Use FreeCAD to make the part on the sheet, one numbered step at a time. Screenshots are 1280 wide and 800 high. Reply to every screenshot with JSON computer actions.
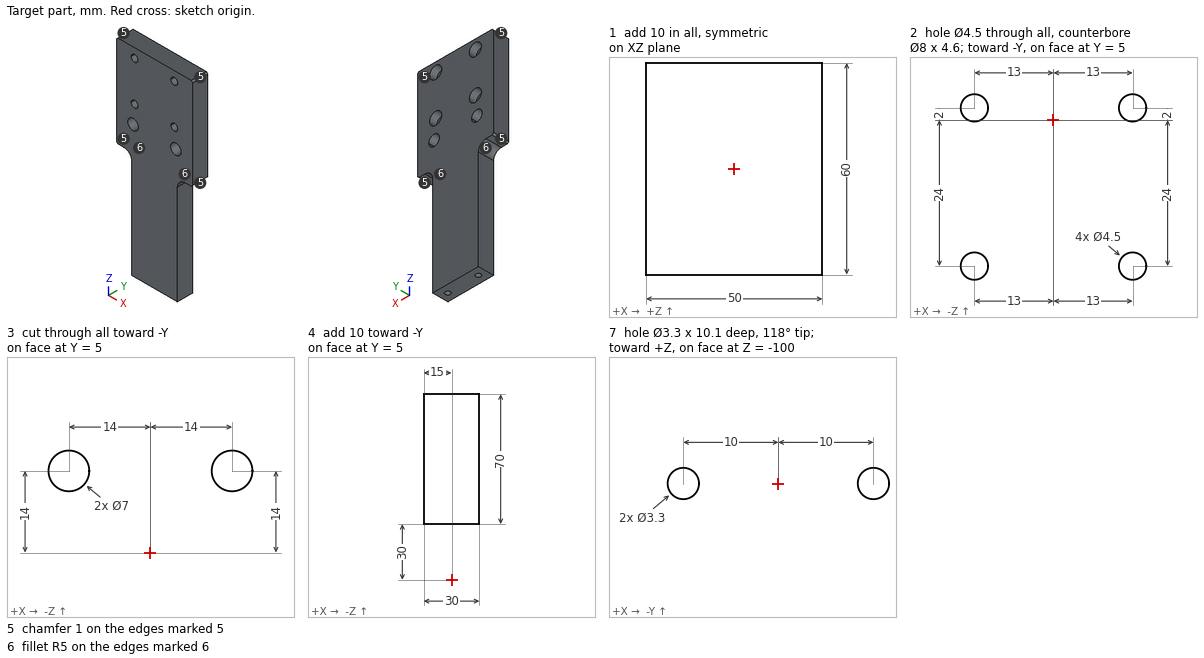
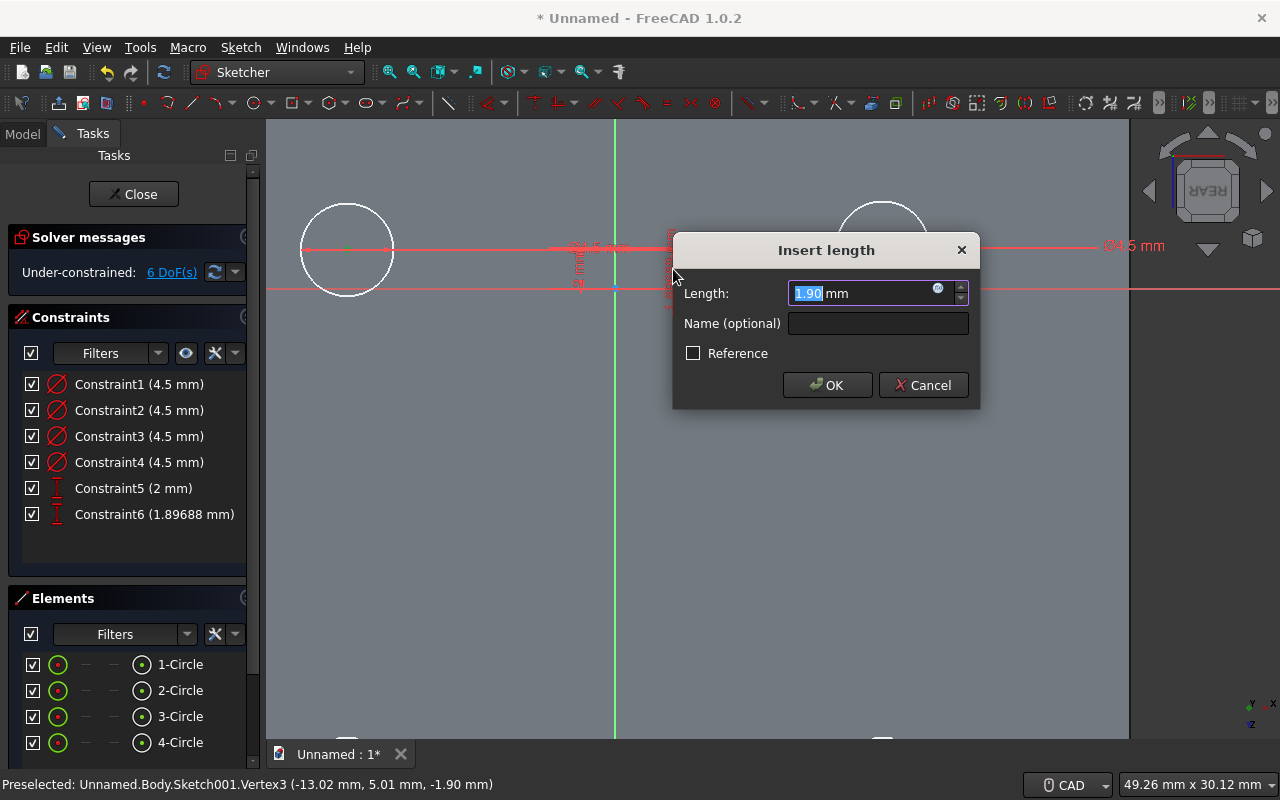
{"action": "type", "text": "2"}
{"action": "key", "text": "Return"}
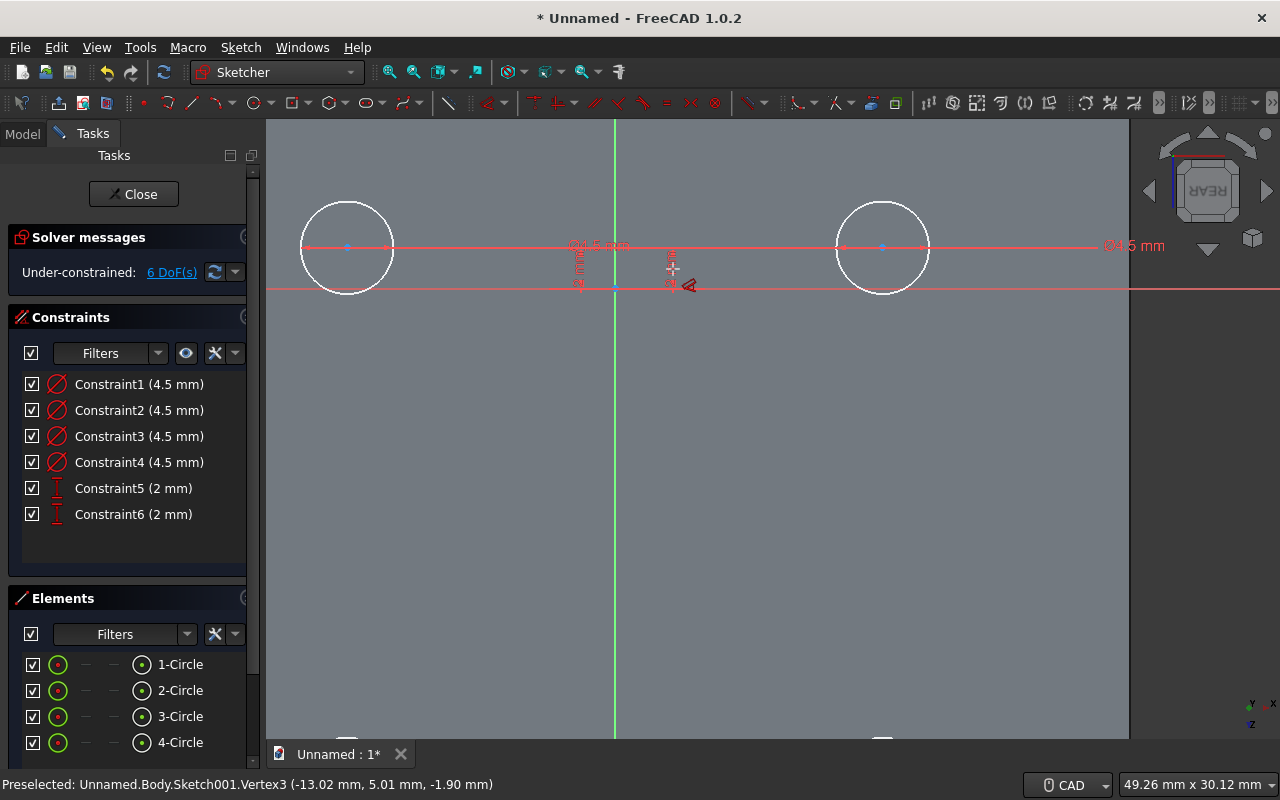
{"action": "scroll", "coordinate": [886, 253], "scroll_direction": "down", "scroll_amount": 2}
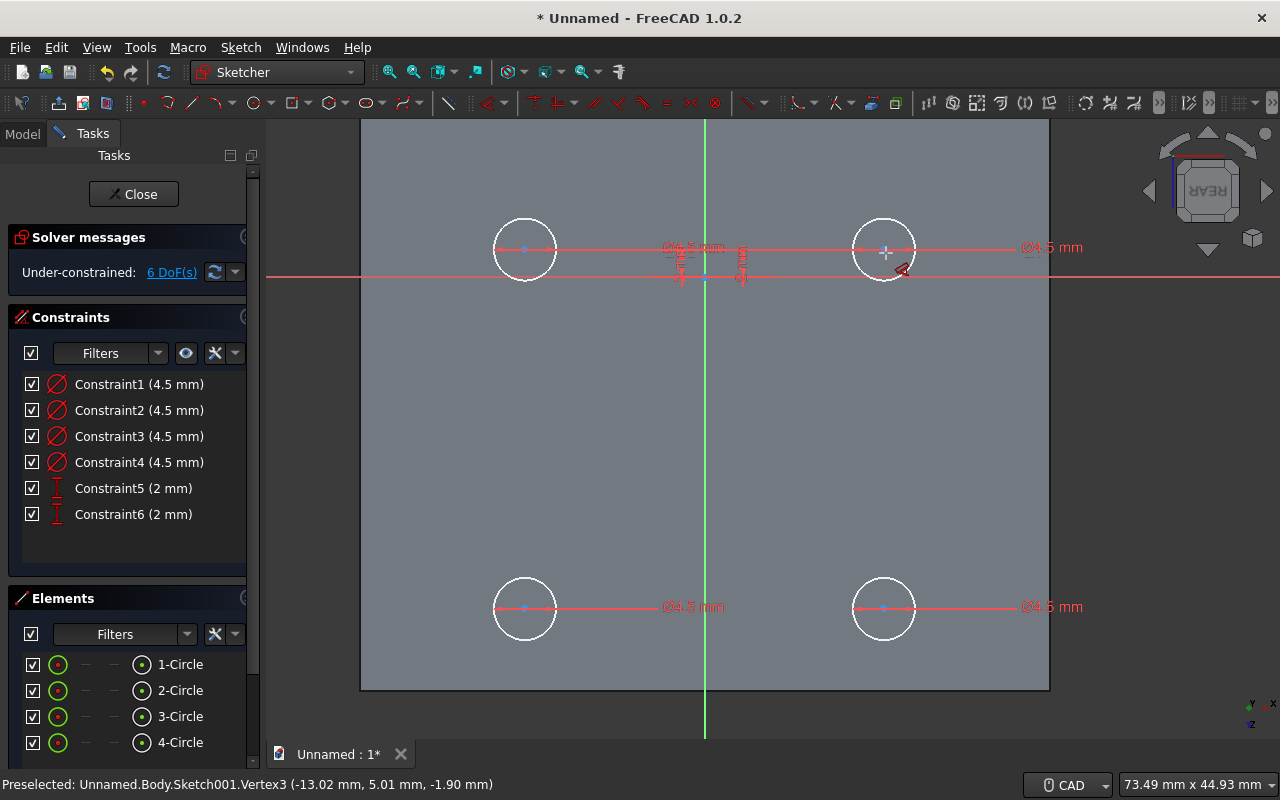
{"action": "left_click", "coordinate": [884, 609]}
{"action": "left_click", "coordinate": [794, 643]}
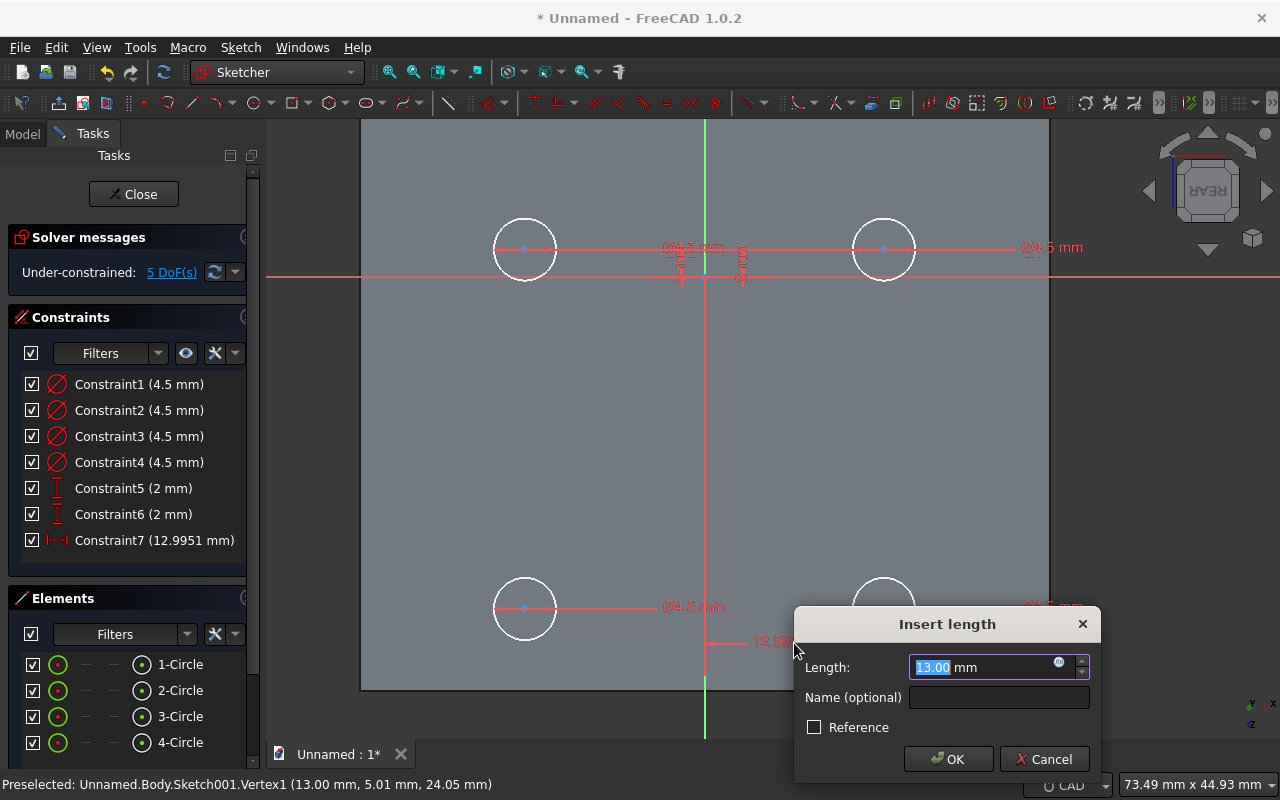
{"action": "type", "text": "13"}
{"action": "key", "text": "Return"}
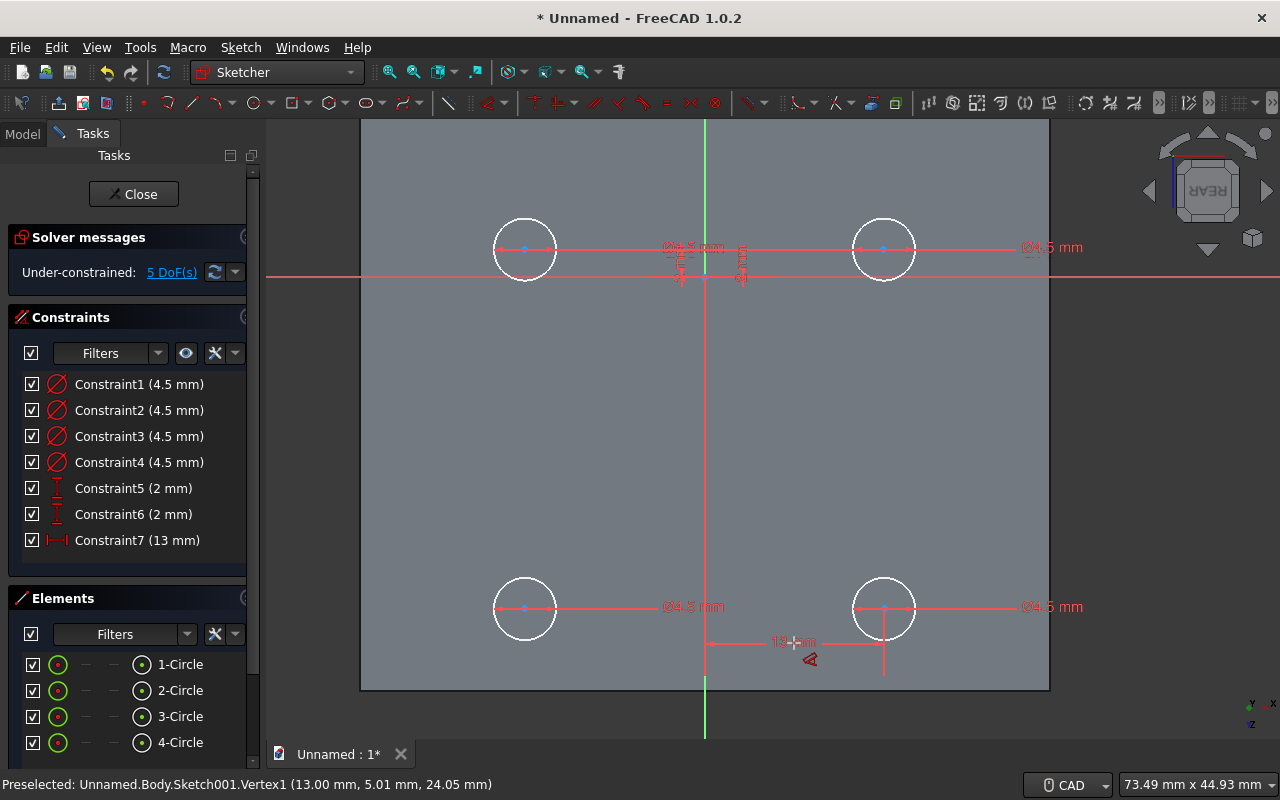
{"action": "left_click", "coordinate": [884, 609]}
{"action": "left_click", "coordinate": [918, 443]}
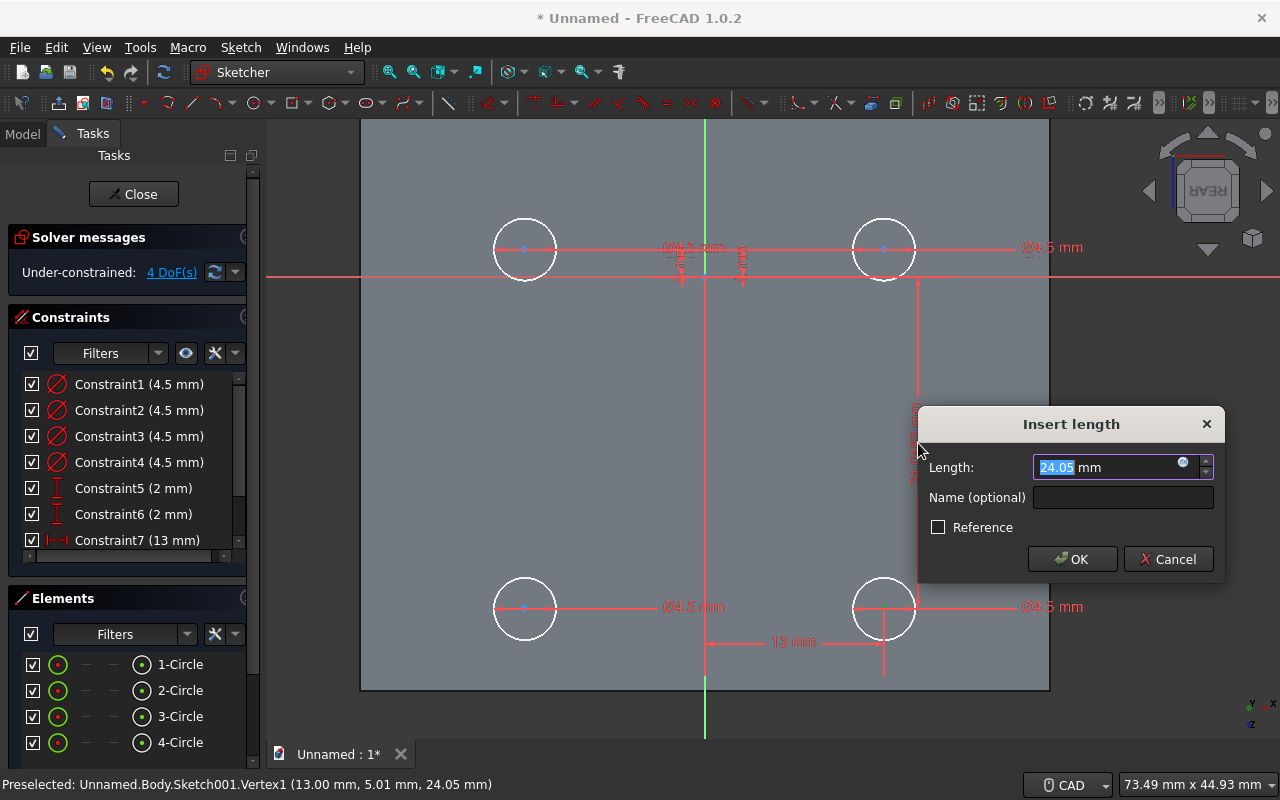
{"action": "type", "text": "24"}
{"action": "key", "text": "Return"}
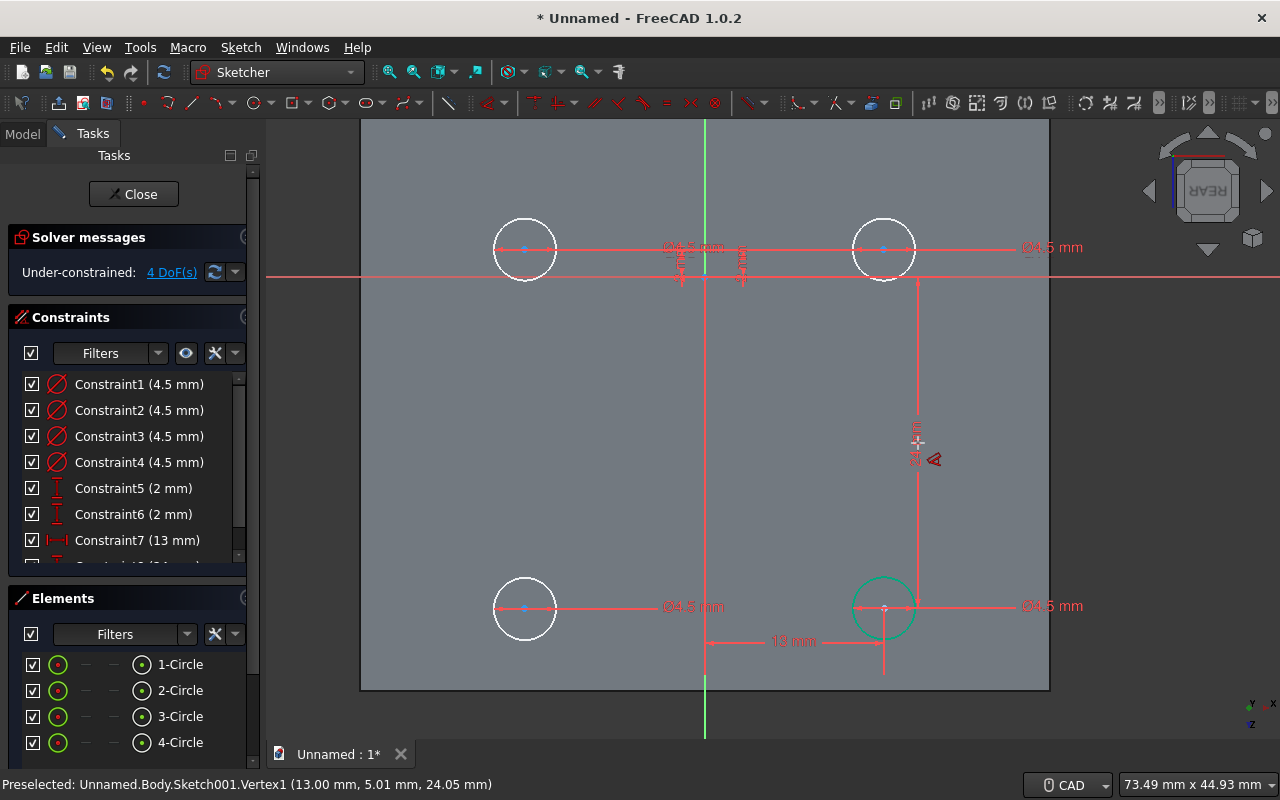
{"action": "left_click", "coordinate": [884, 250]}
{"action": "left_click", "coordinate": [794, 216]}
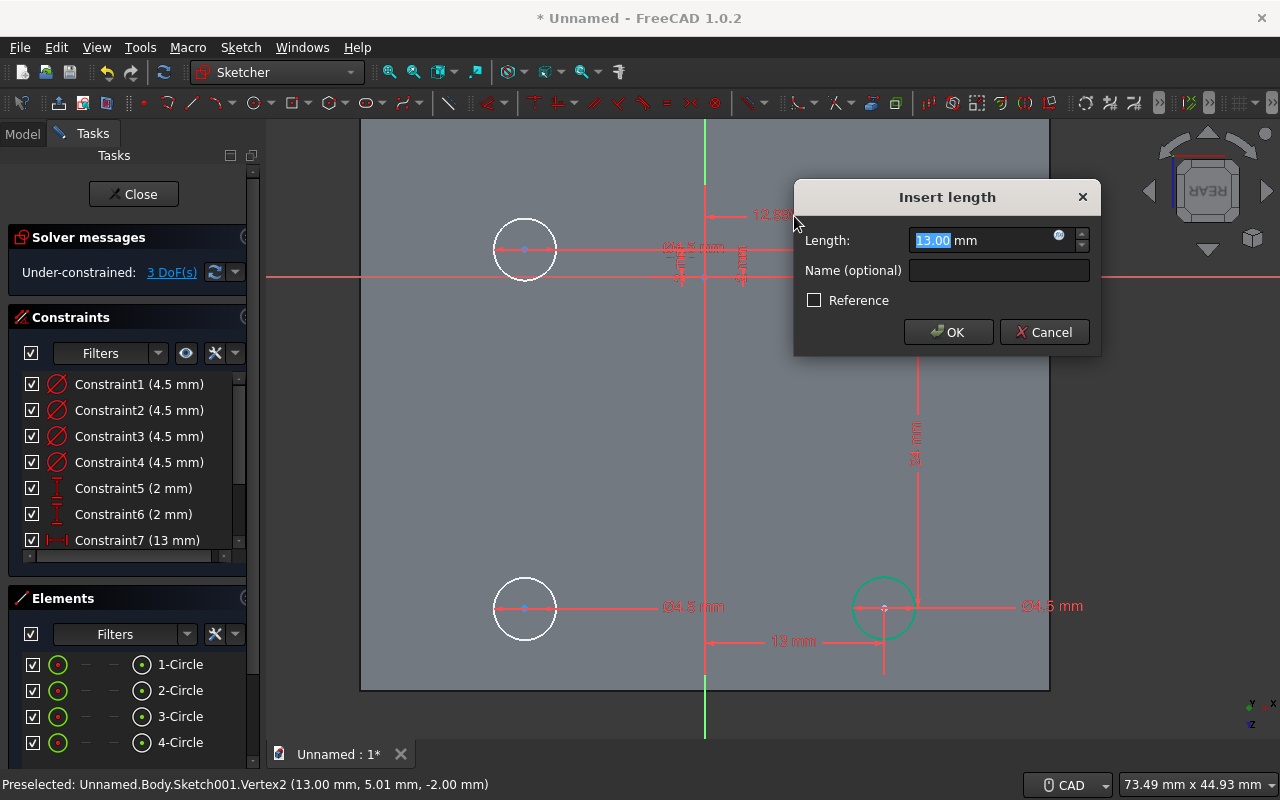
{"action": "type", "text": "13"}
{"action": "key", "text": "Return"}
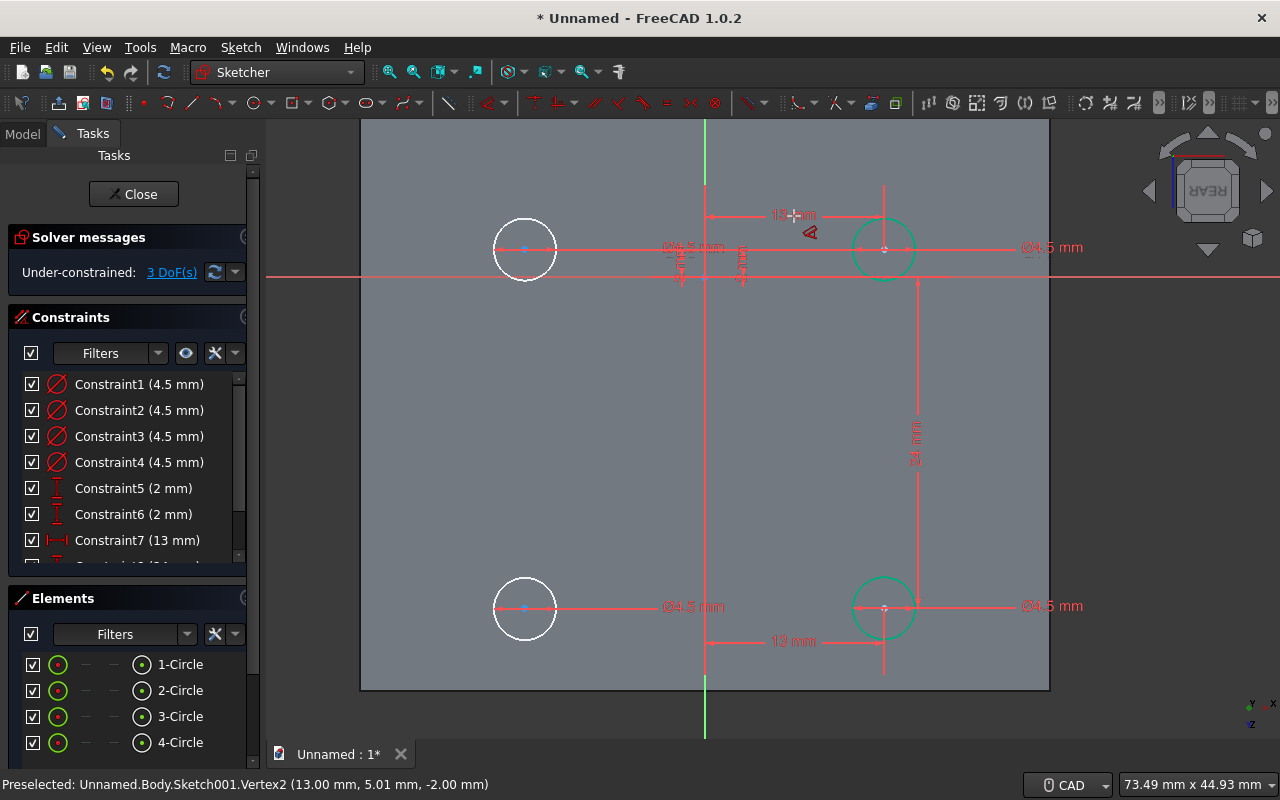
{"action": "left_click", "coordinate": [525, 250]}
{"action": "left_click", "coordinate": [615, 216]}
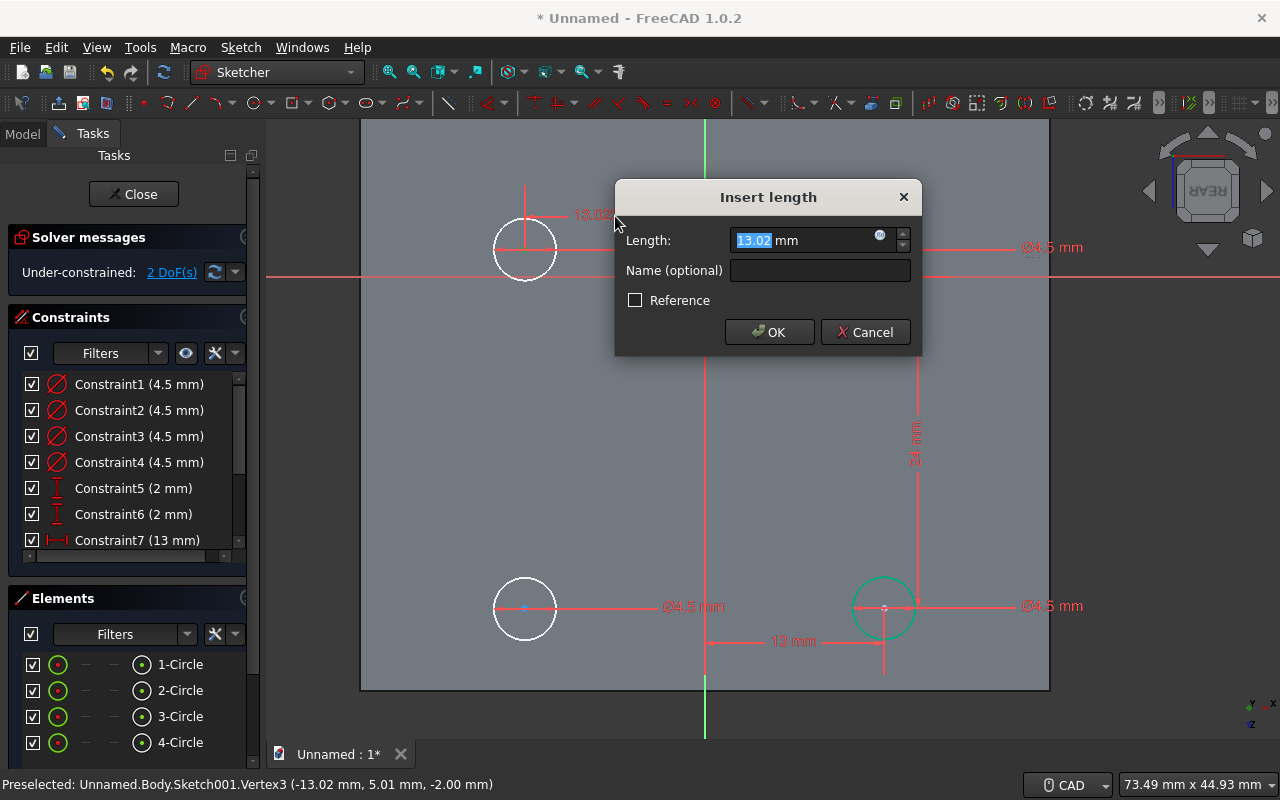
{"action": "type", "text": "13"}
{"action": "key", "text": "Return"}